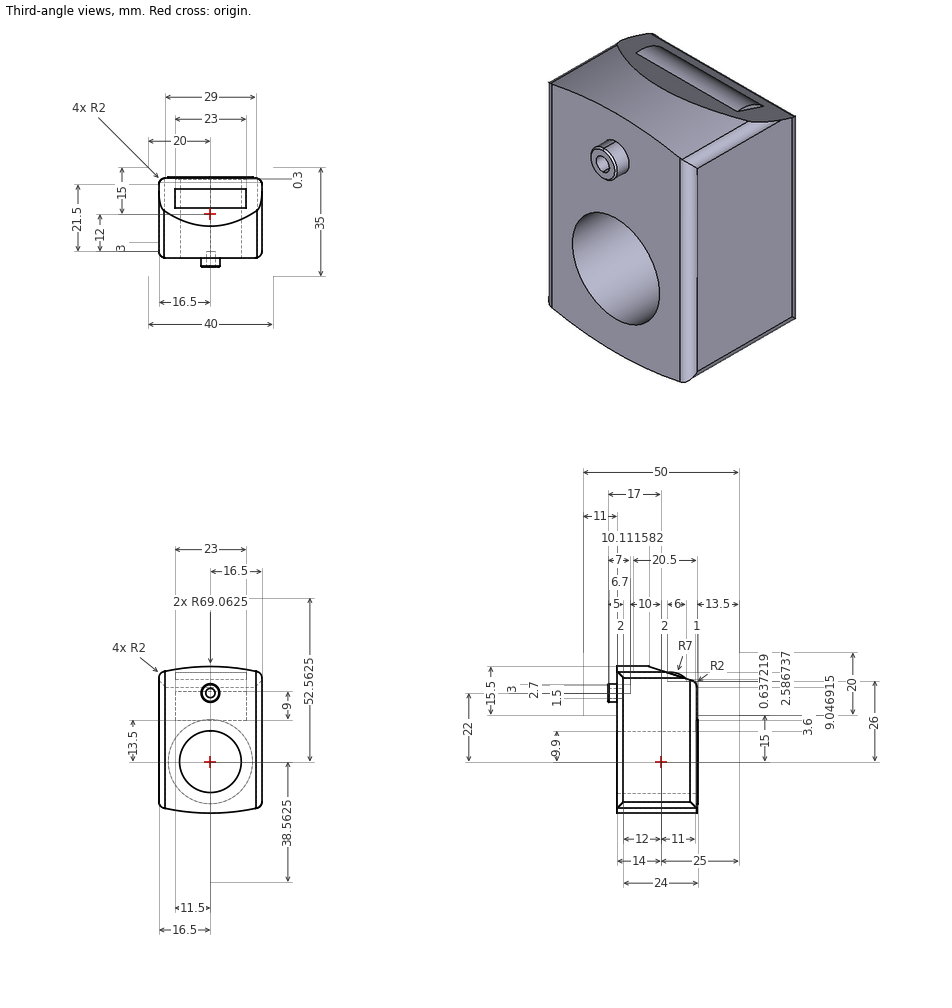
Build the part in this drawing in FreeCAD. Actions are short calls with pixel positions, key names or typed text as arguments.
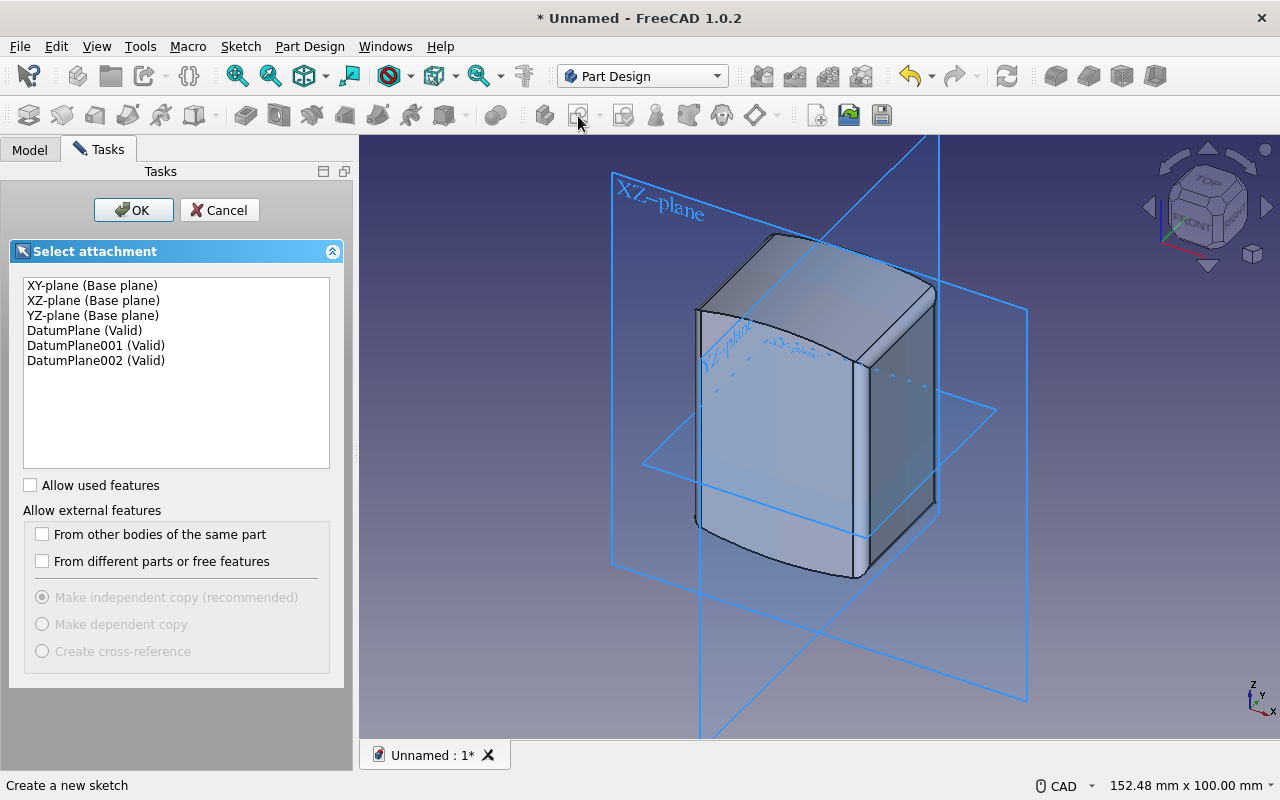
click(84, 316)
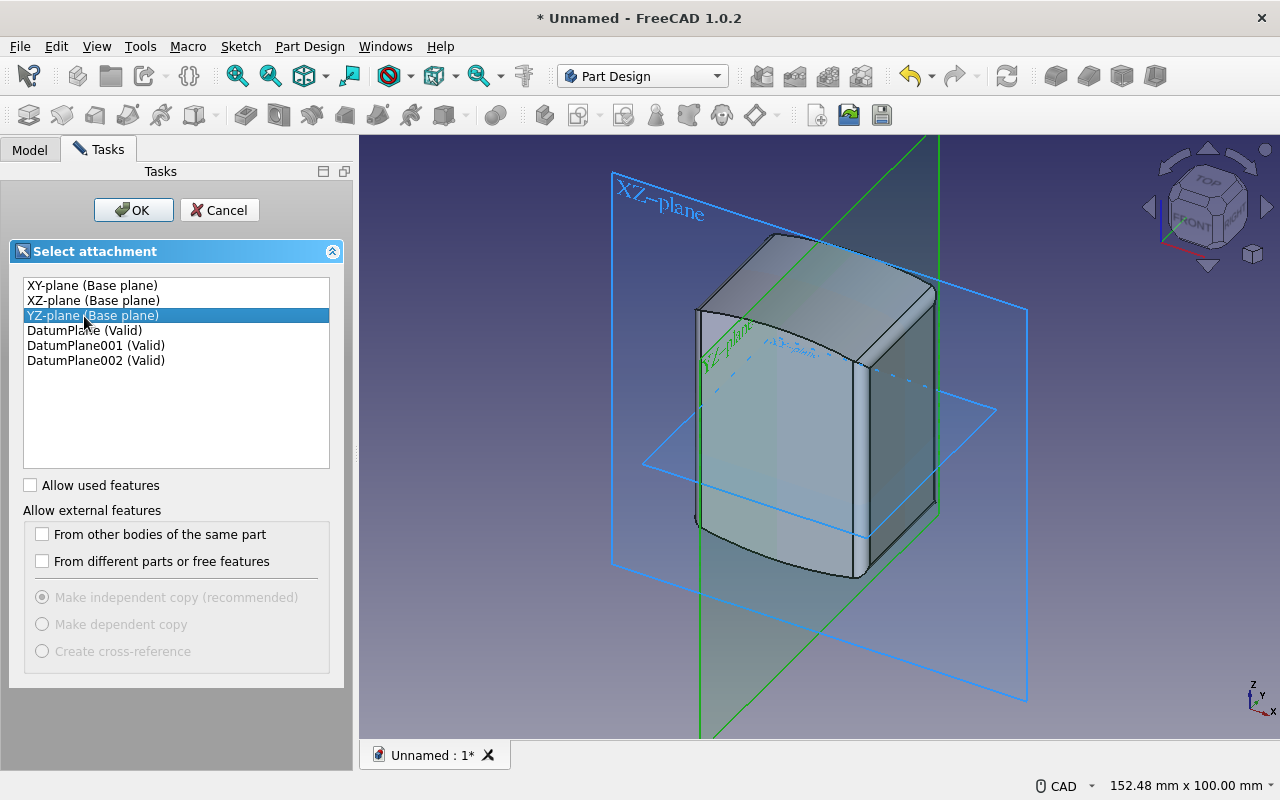
click(134, 210)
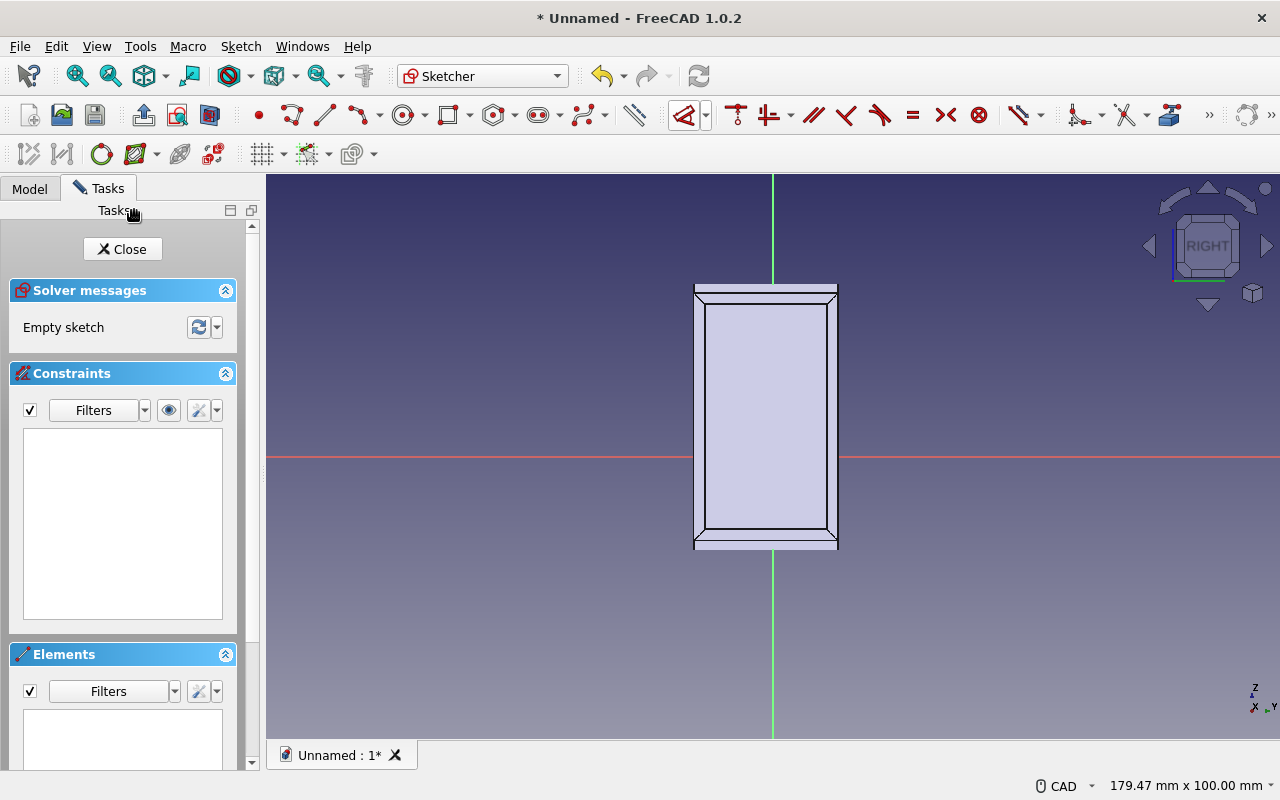
click(210, 116)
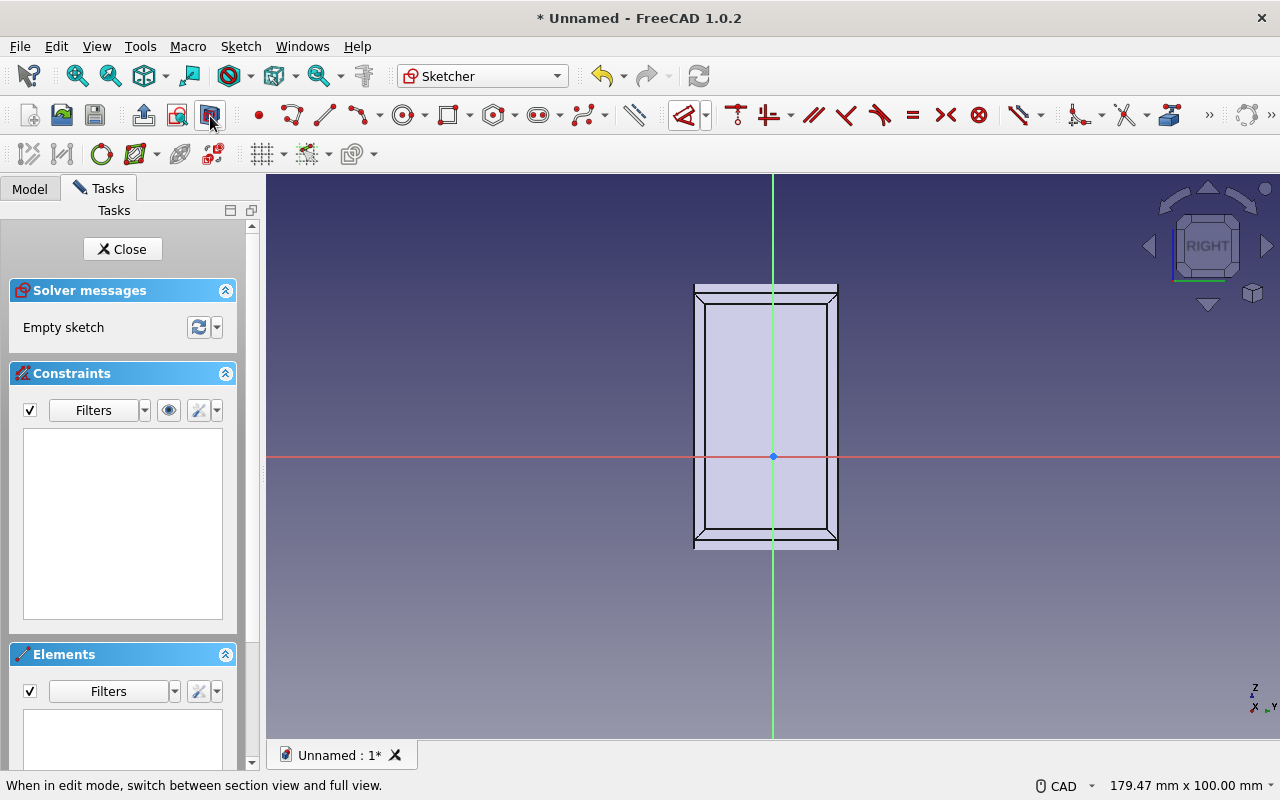
scroll(795, 419, up, 7)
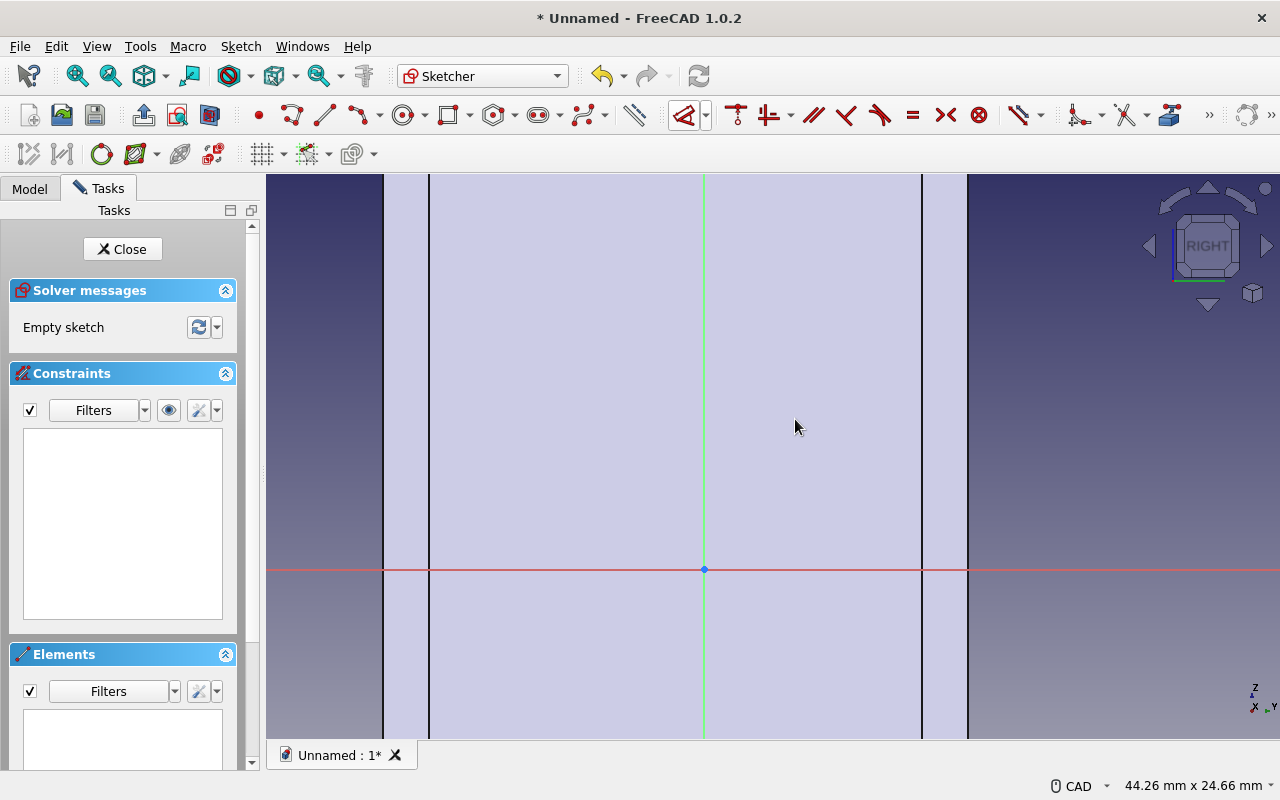
click(448, 116)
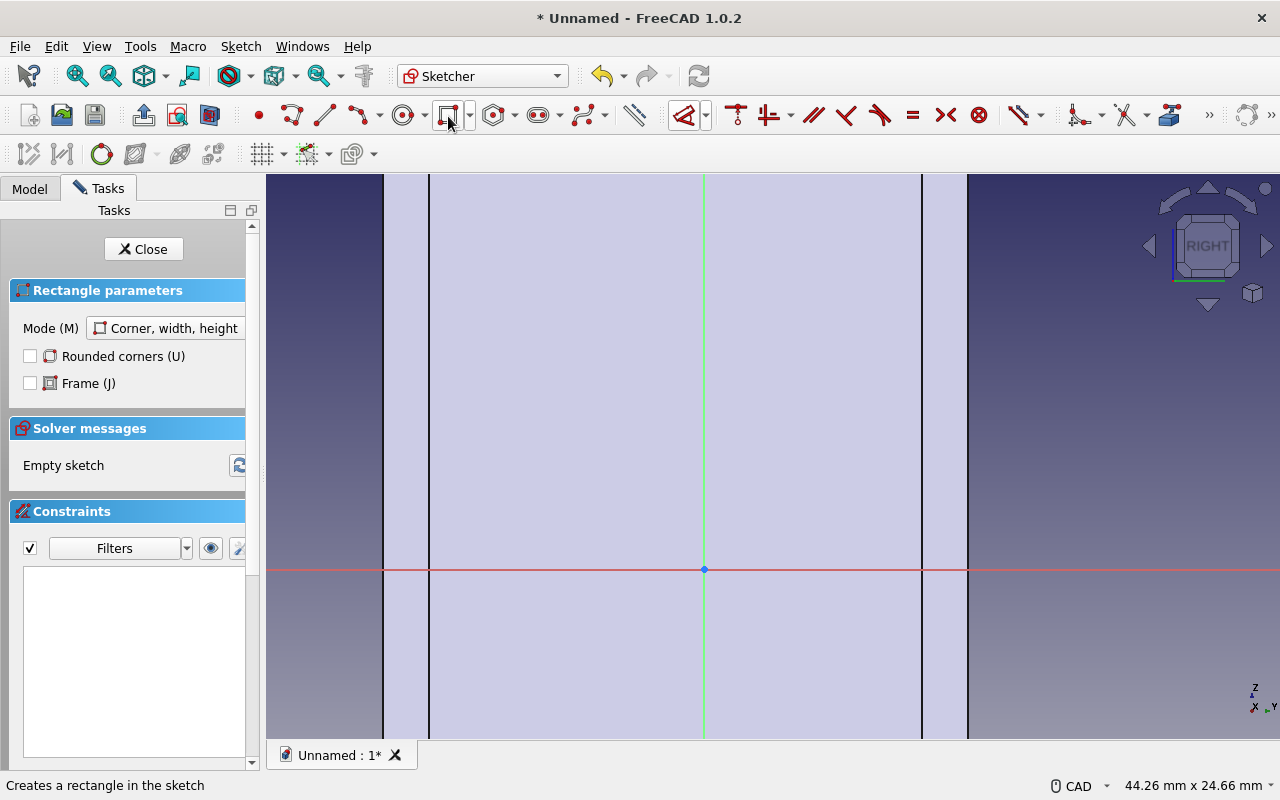
click(429, 343)
click(979, 570)
key(Escape)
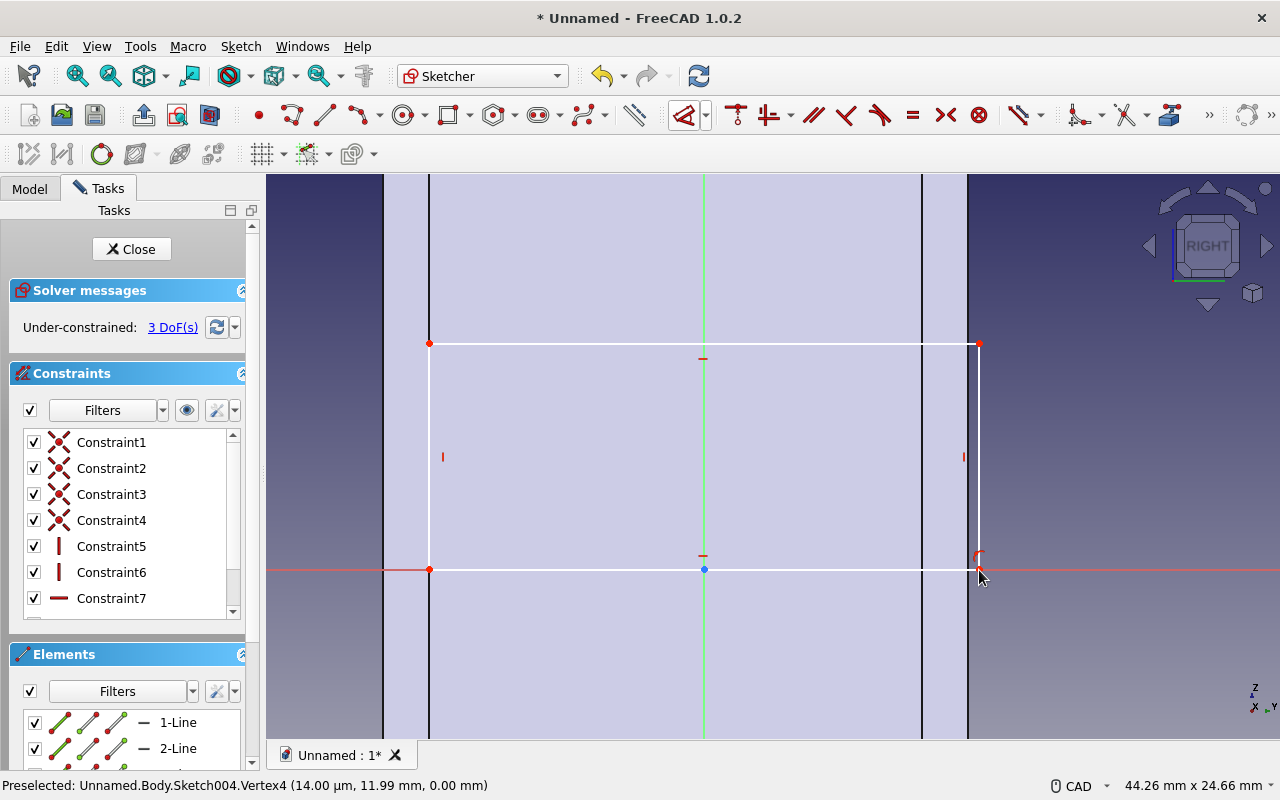
click(594, 570)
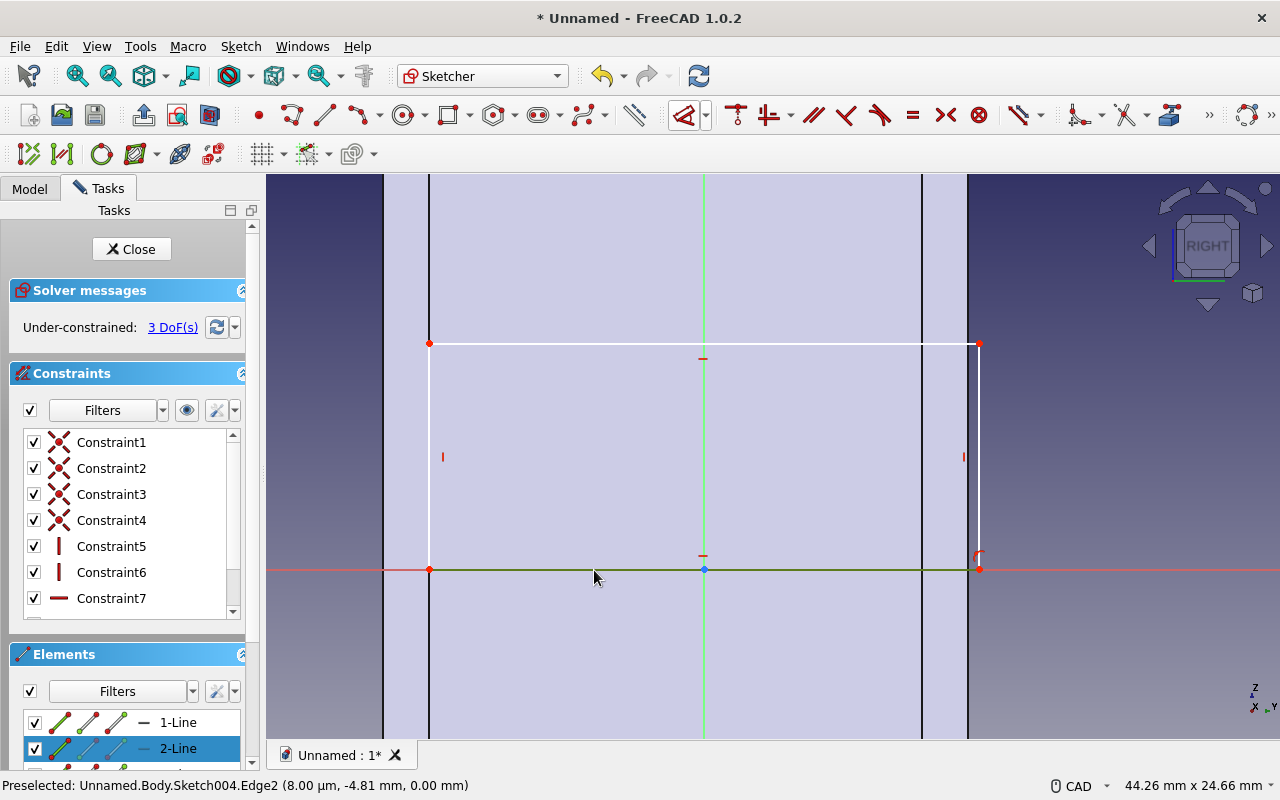
key(l)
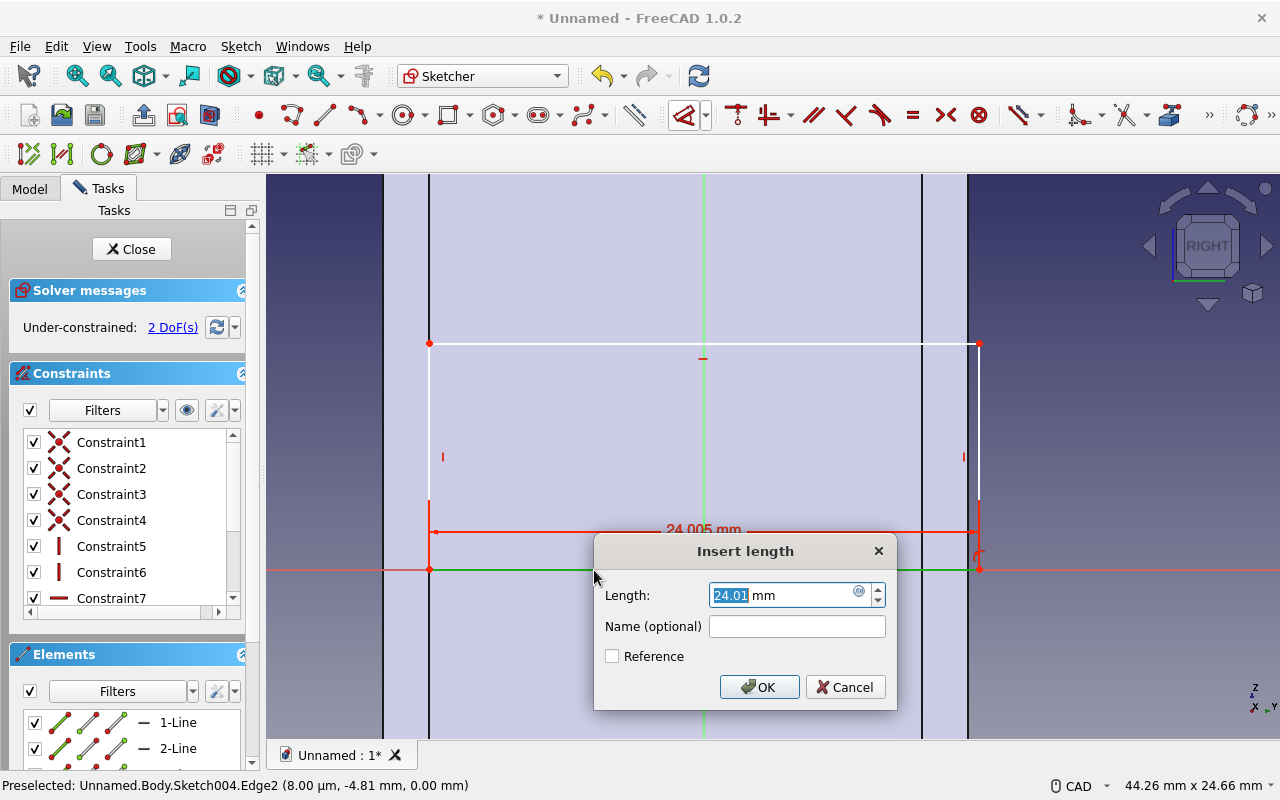
text(24)
key(Return)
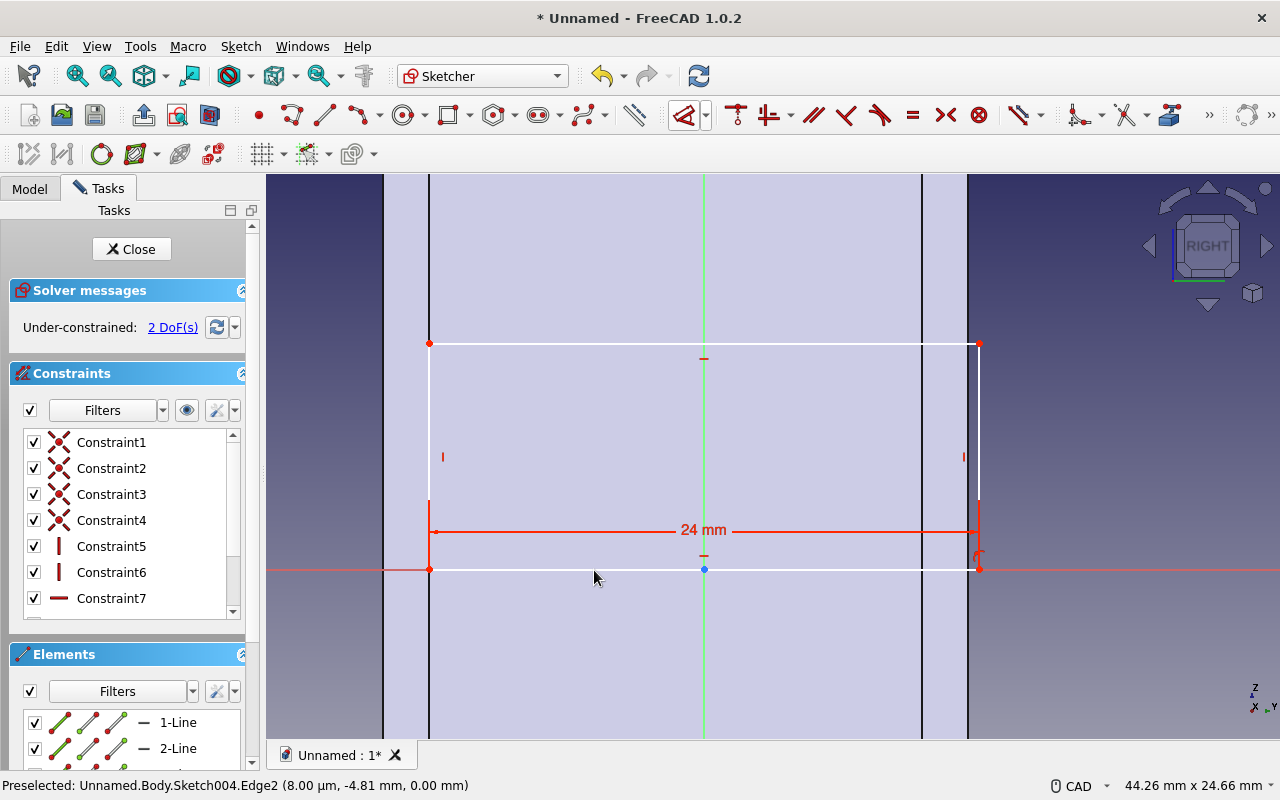
click(429, 412)